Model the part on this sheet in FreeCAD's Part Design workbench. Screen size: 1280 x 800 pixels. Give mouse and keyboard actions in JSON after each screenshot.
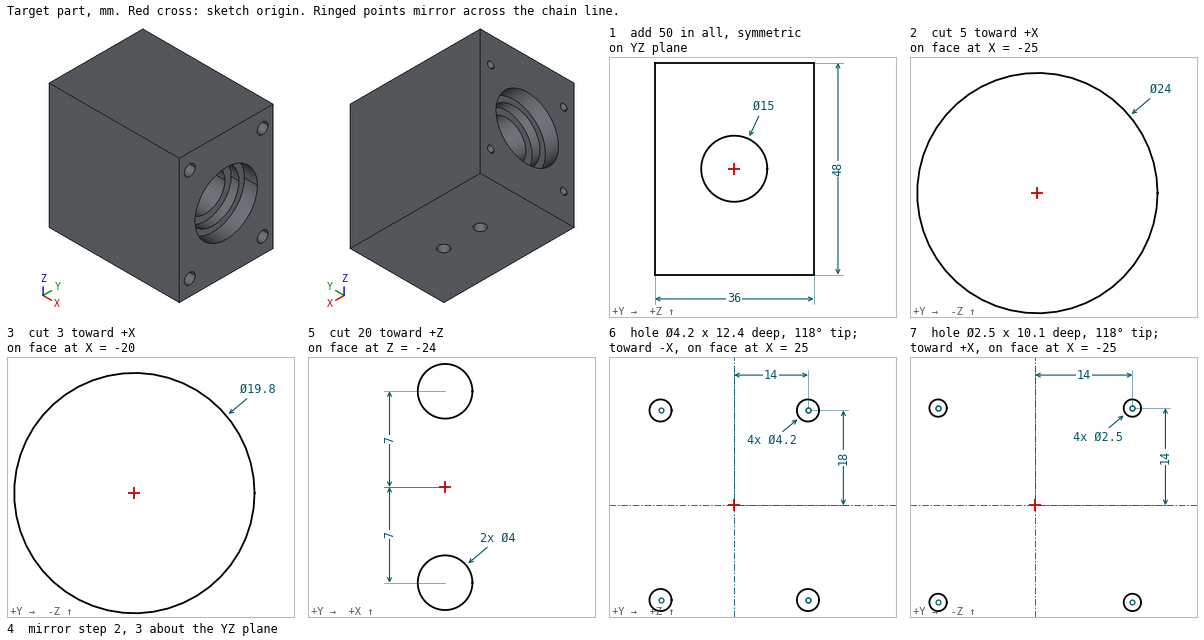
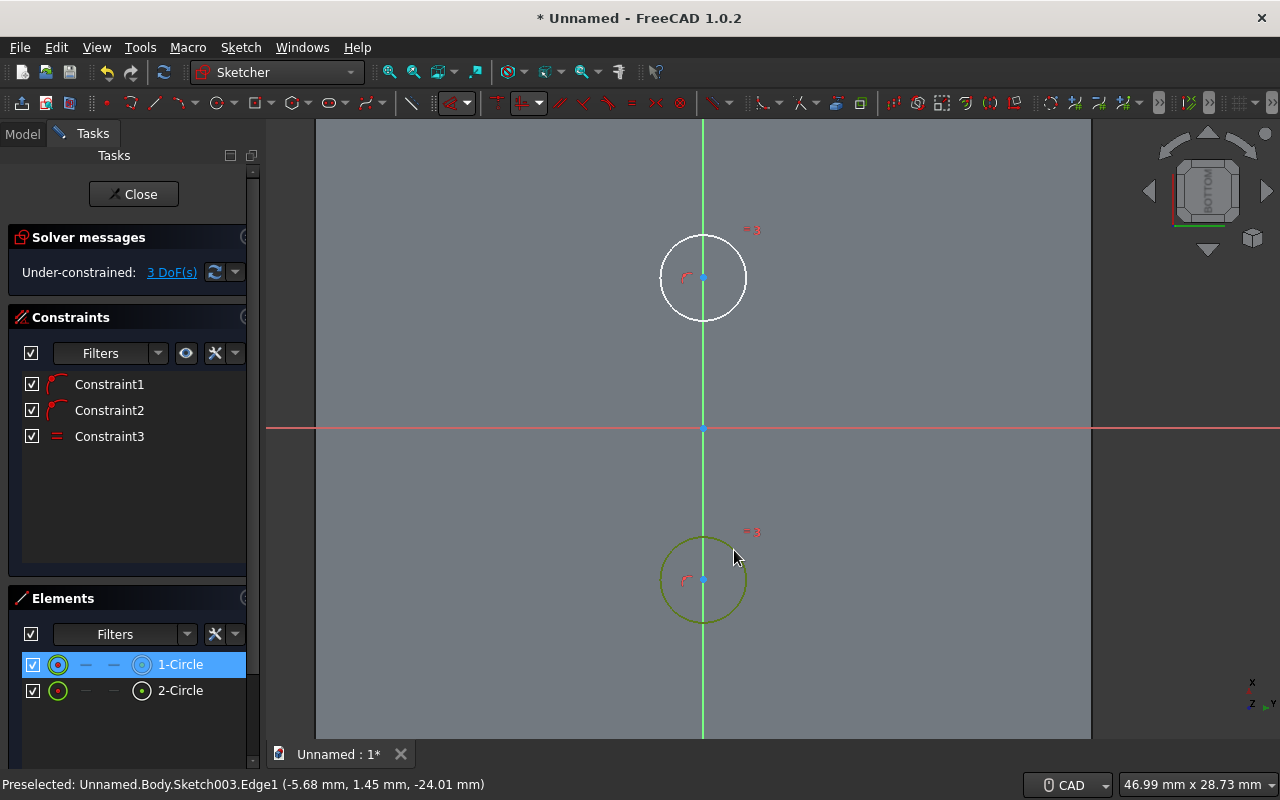
{"action": "key", "text": "k o"}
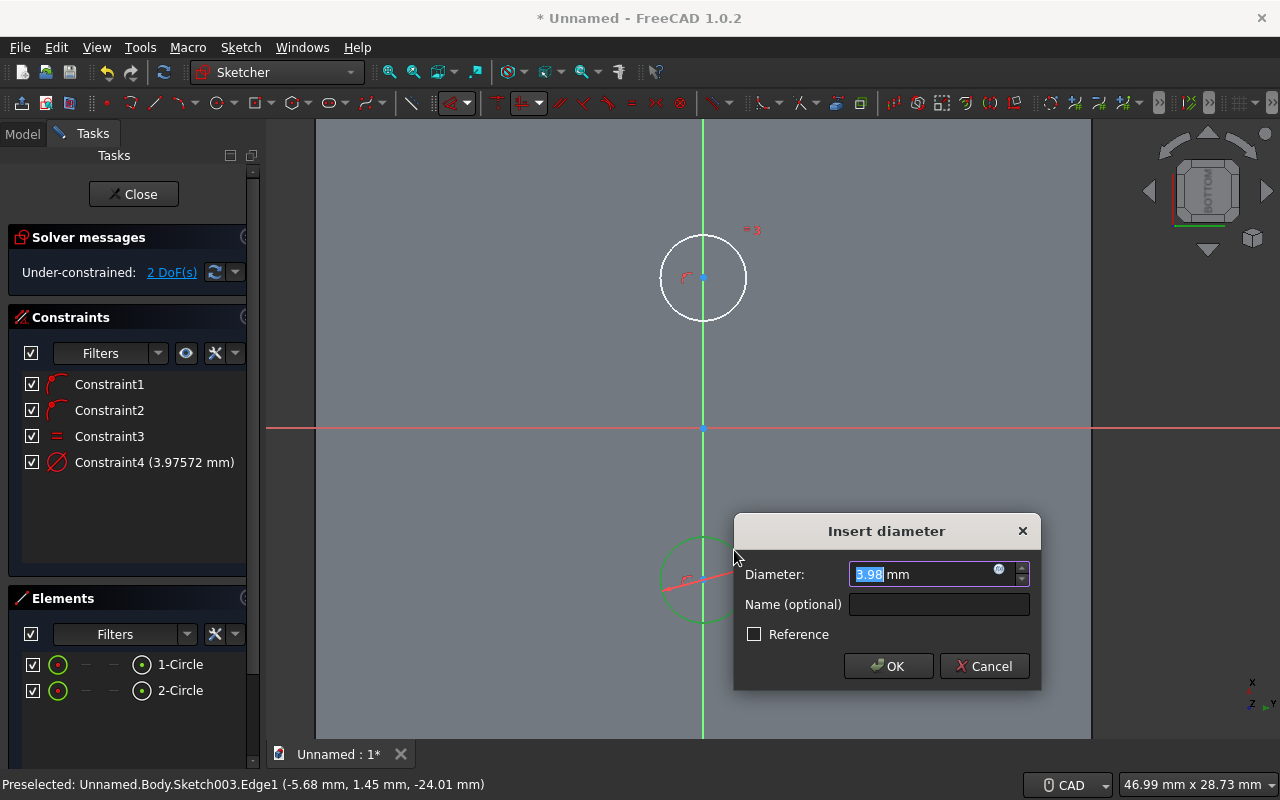
{"action": "type", "text": "4"}
{"action": "key", "text": "Return"}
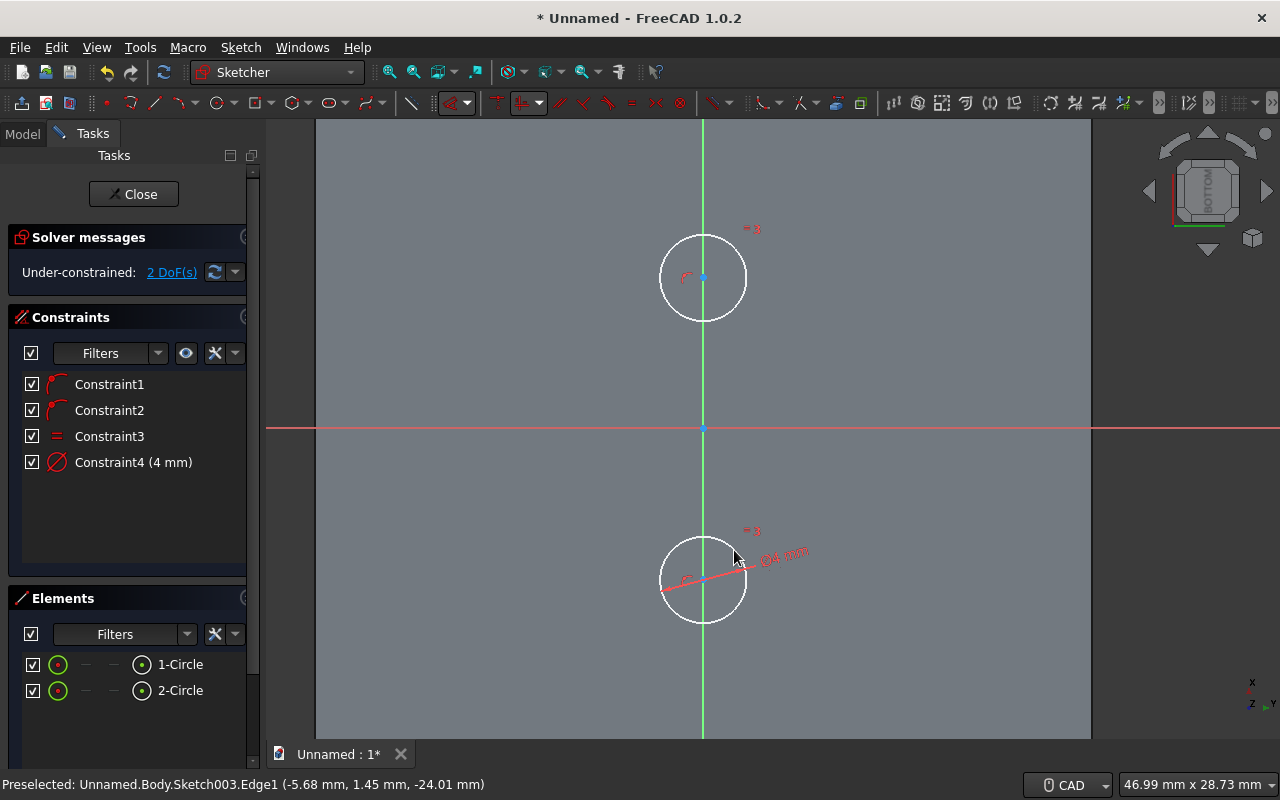
{"action": "left_click", "coordinate": [703, 580]}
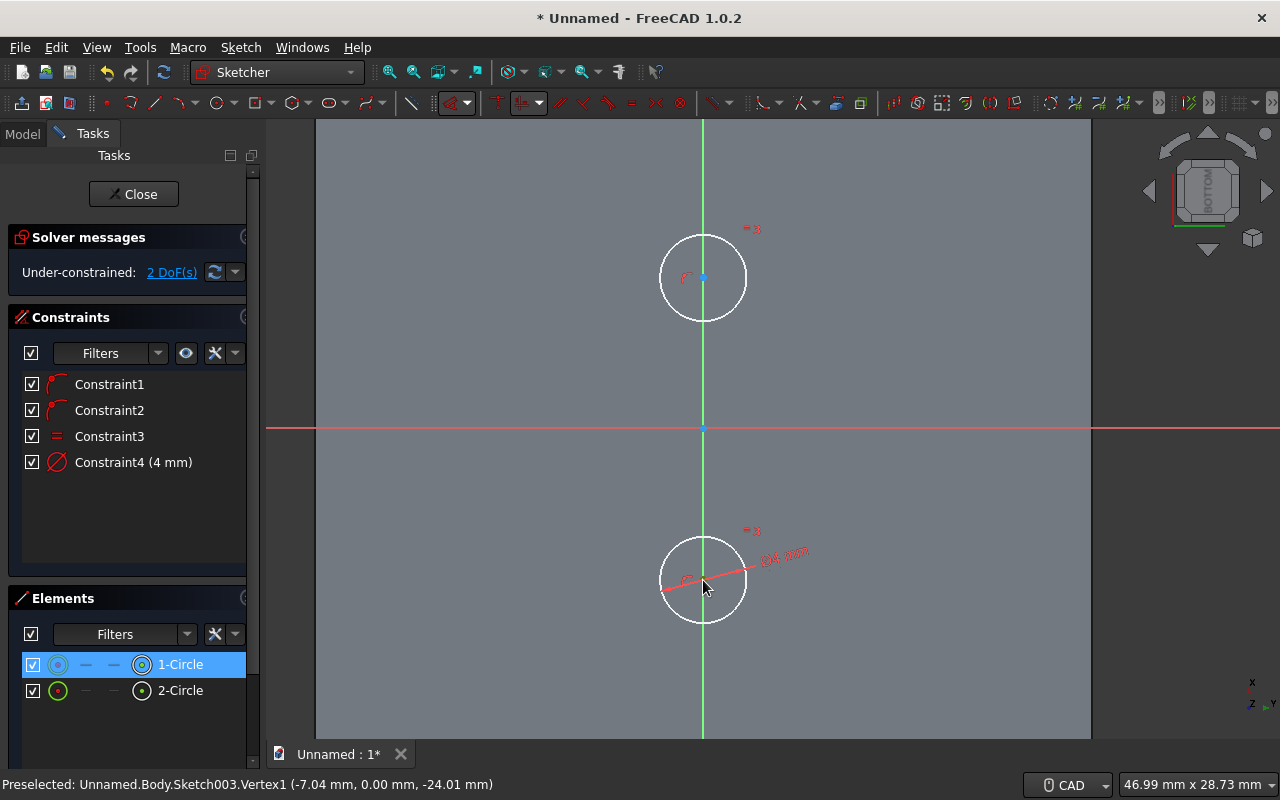
{"action": "key", "text": "i"}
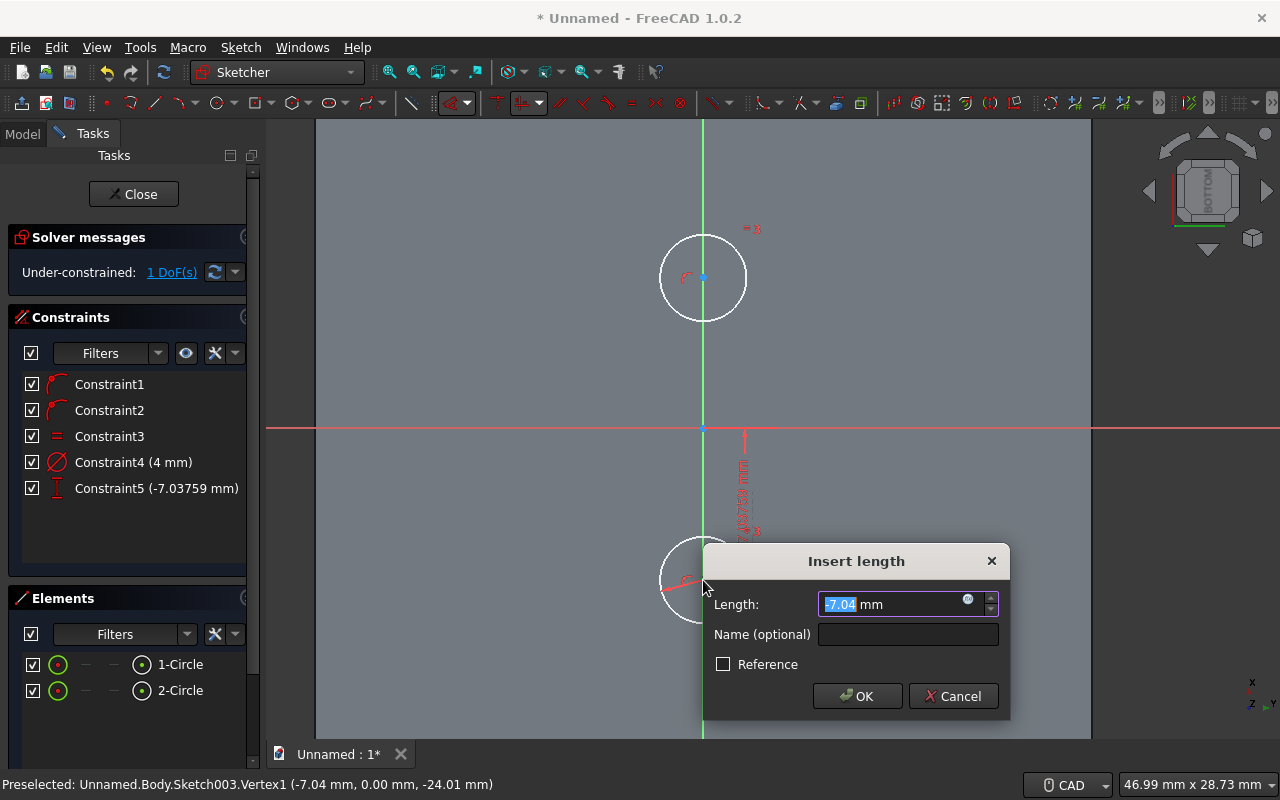
{"action": "type", "text": "-7"}
{"action": "key", "text": "Return"}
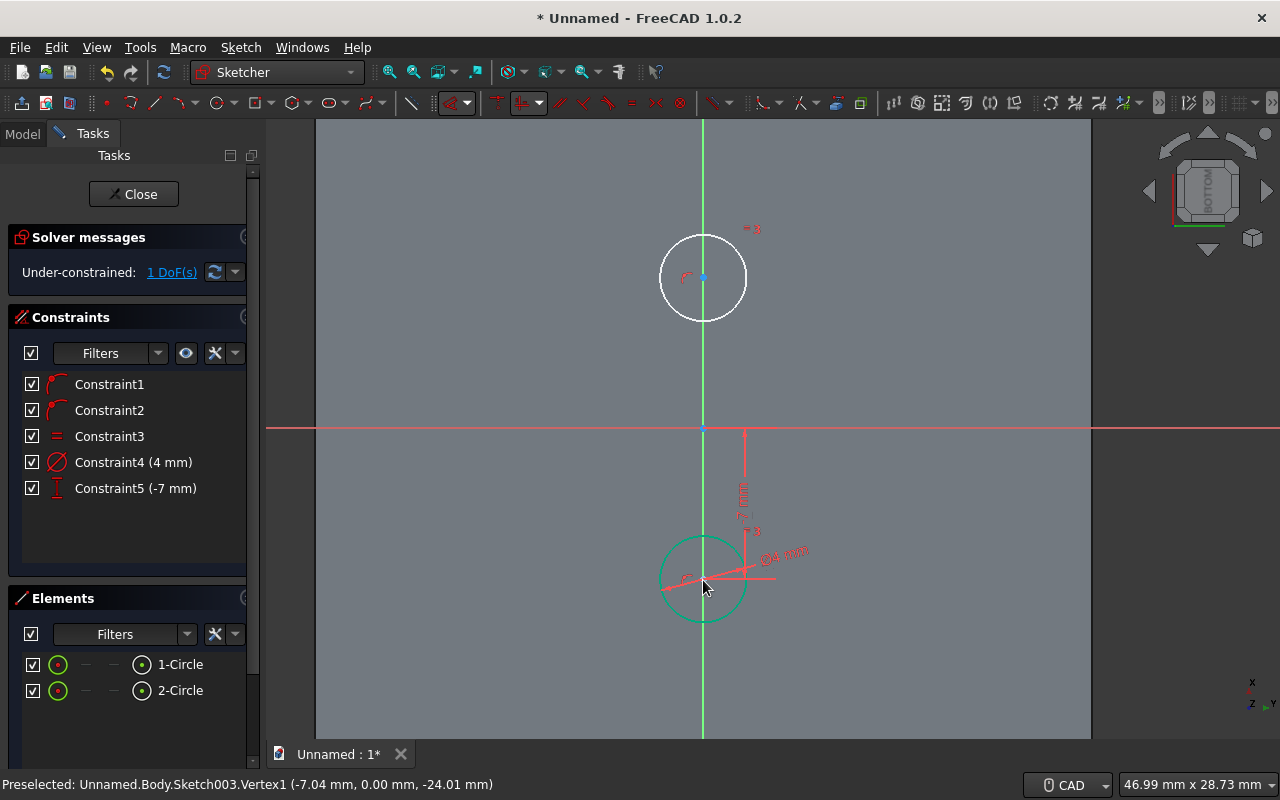
{"action": "left_click", "coordinate": [703, 278]}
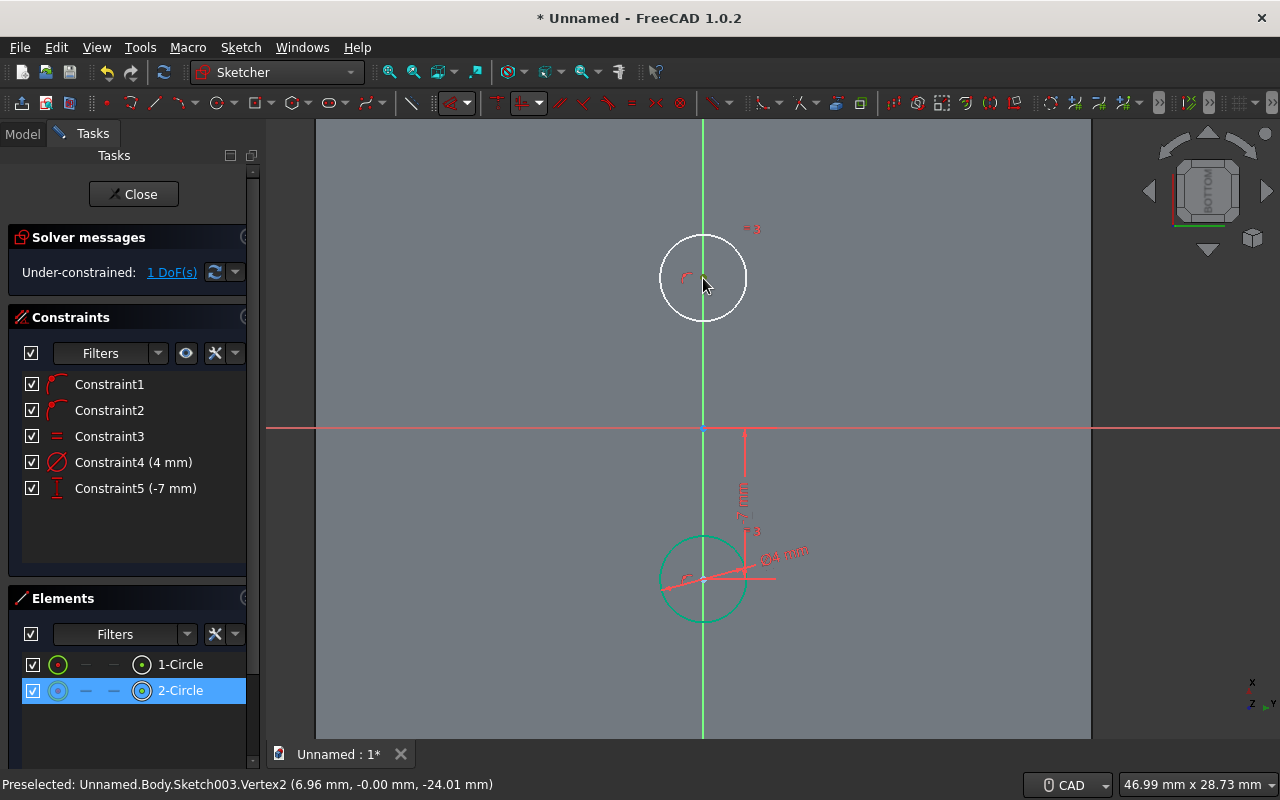
{"action": "key", "text": "i"}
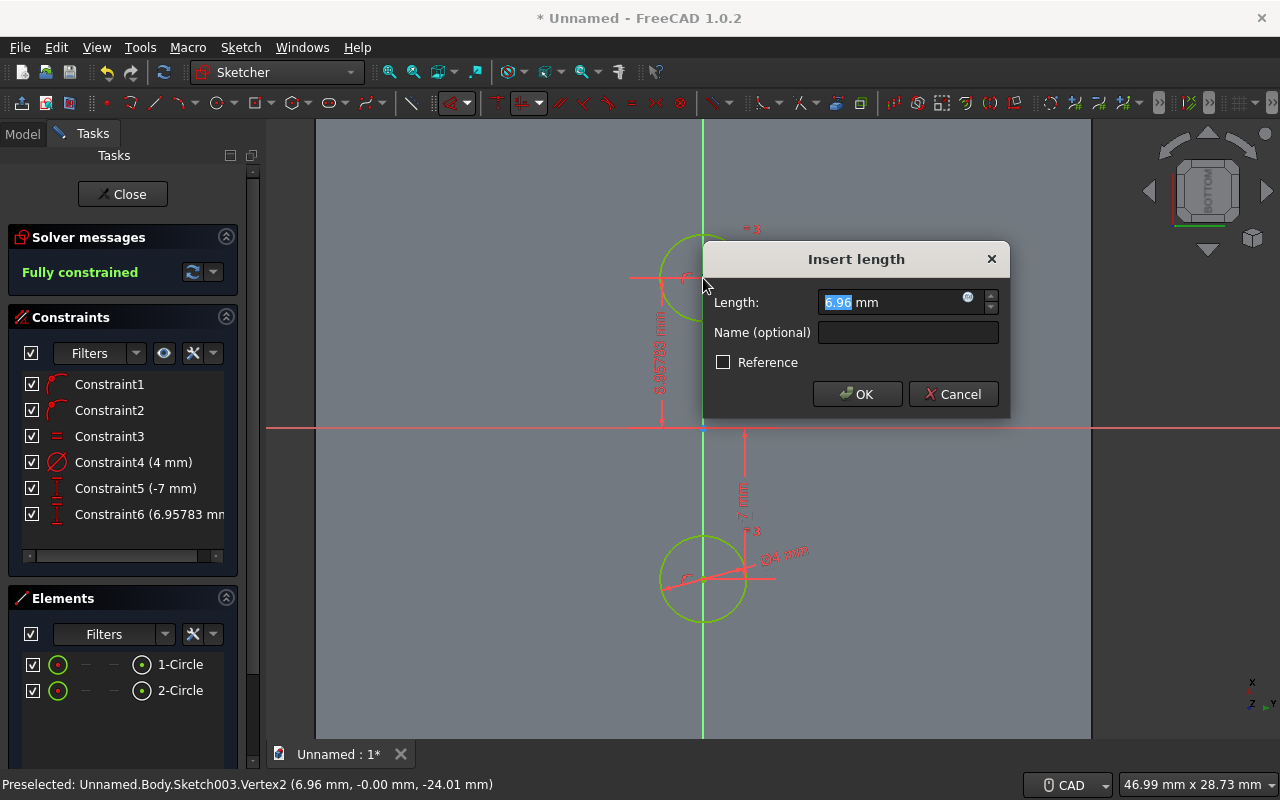
{"action": "type", "text": "7"}
{"action": "key", "text": "Return"}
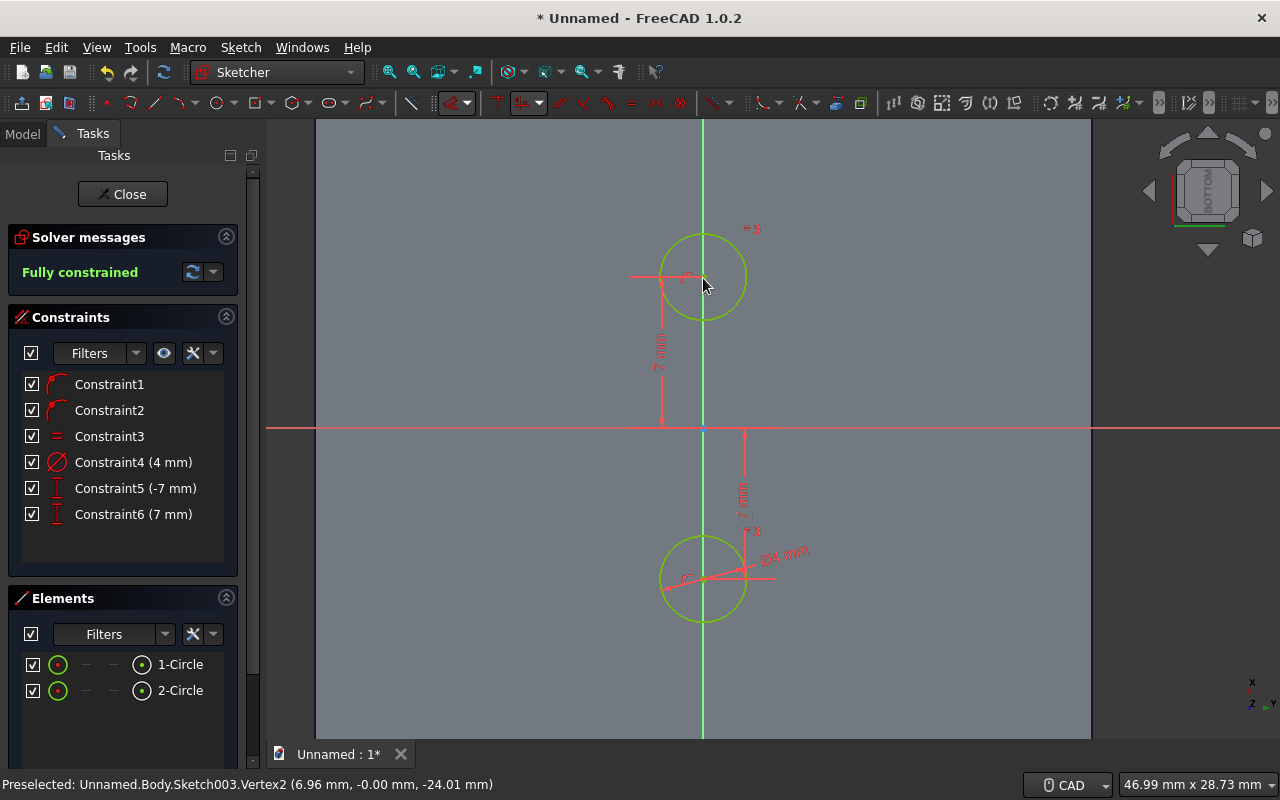
{"action": "left_click", "coordinate": [123, 194]}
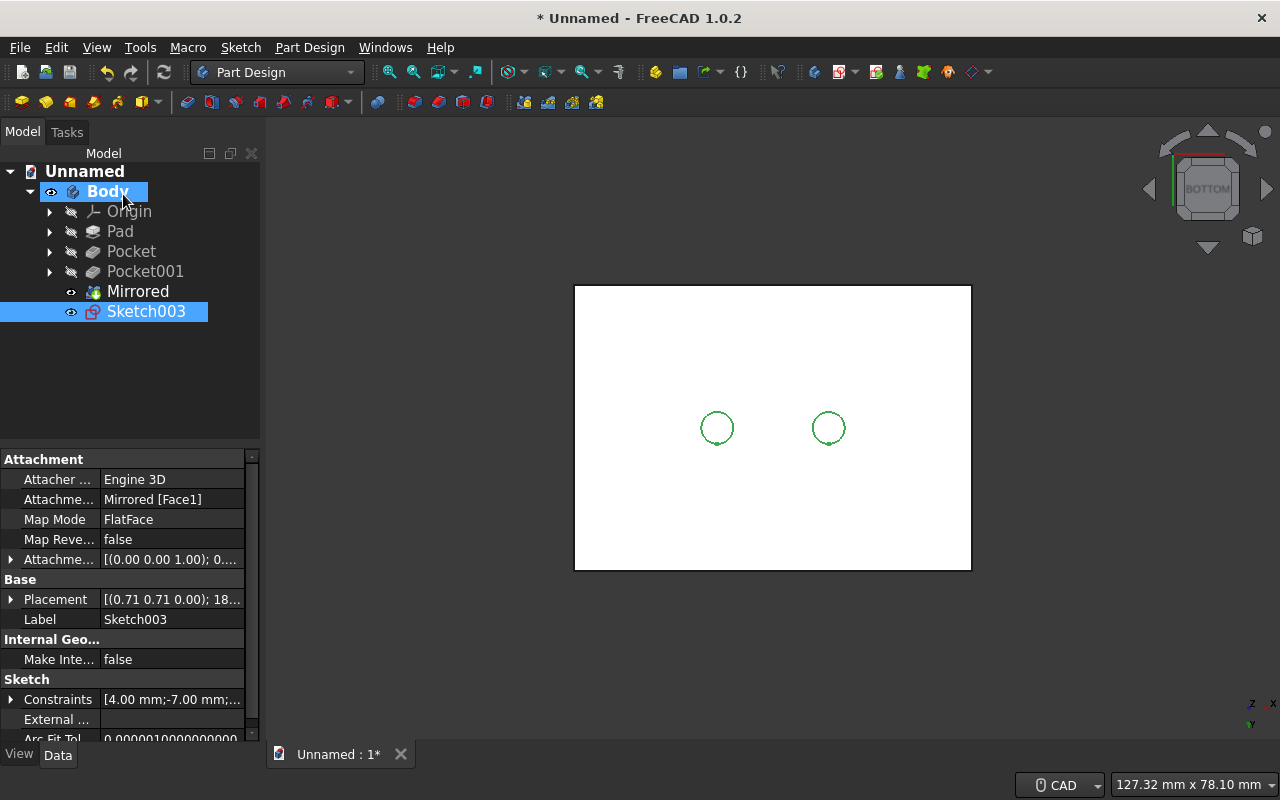
{"action": "left_click", "coordinate": [188, 102]}